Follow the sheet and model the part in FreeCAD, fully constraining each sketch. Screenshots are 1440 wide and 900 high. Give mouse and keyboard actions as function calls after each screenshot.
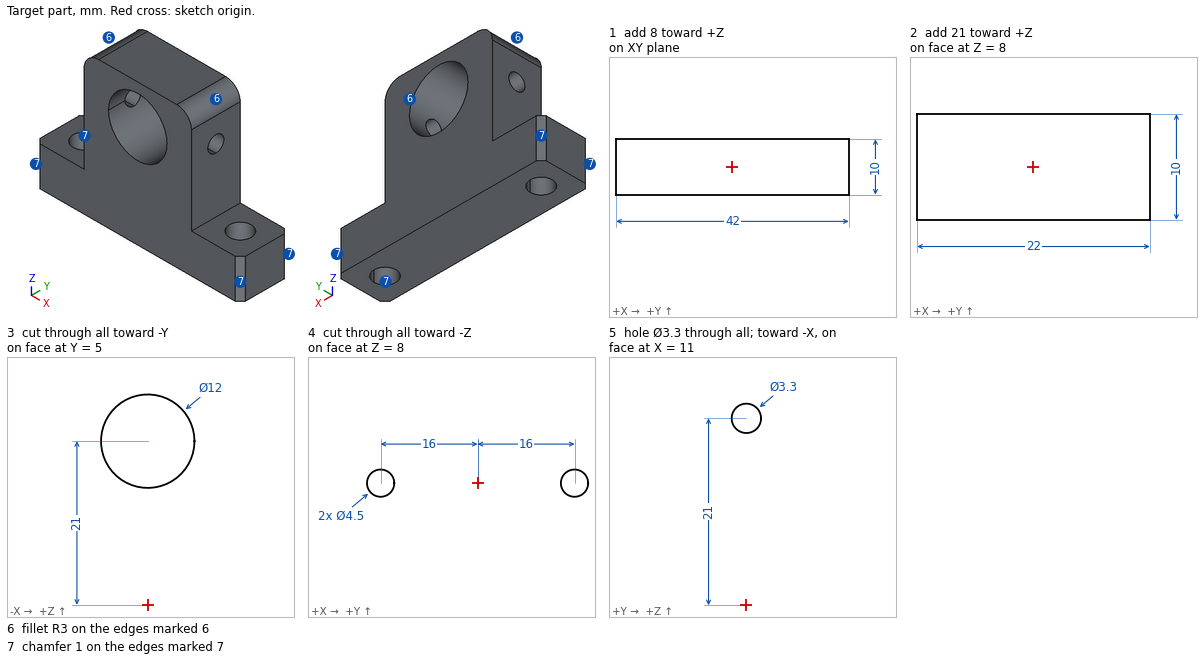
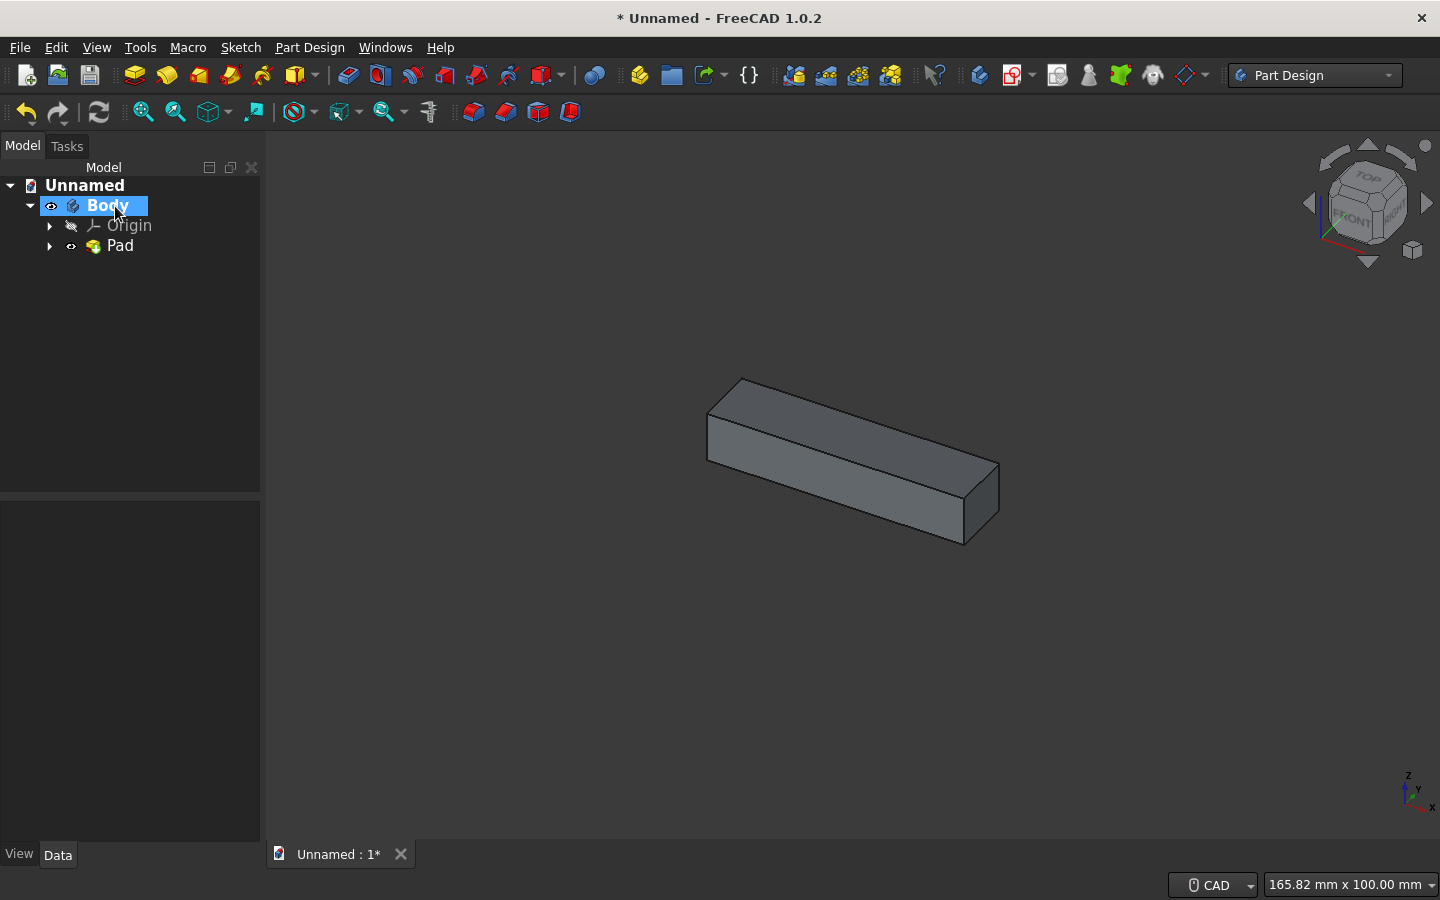
key(v)
key(f)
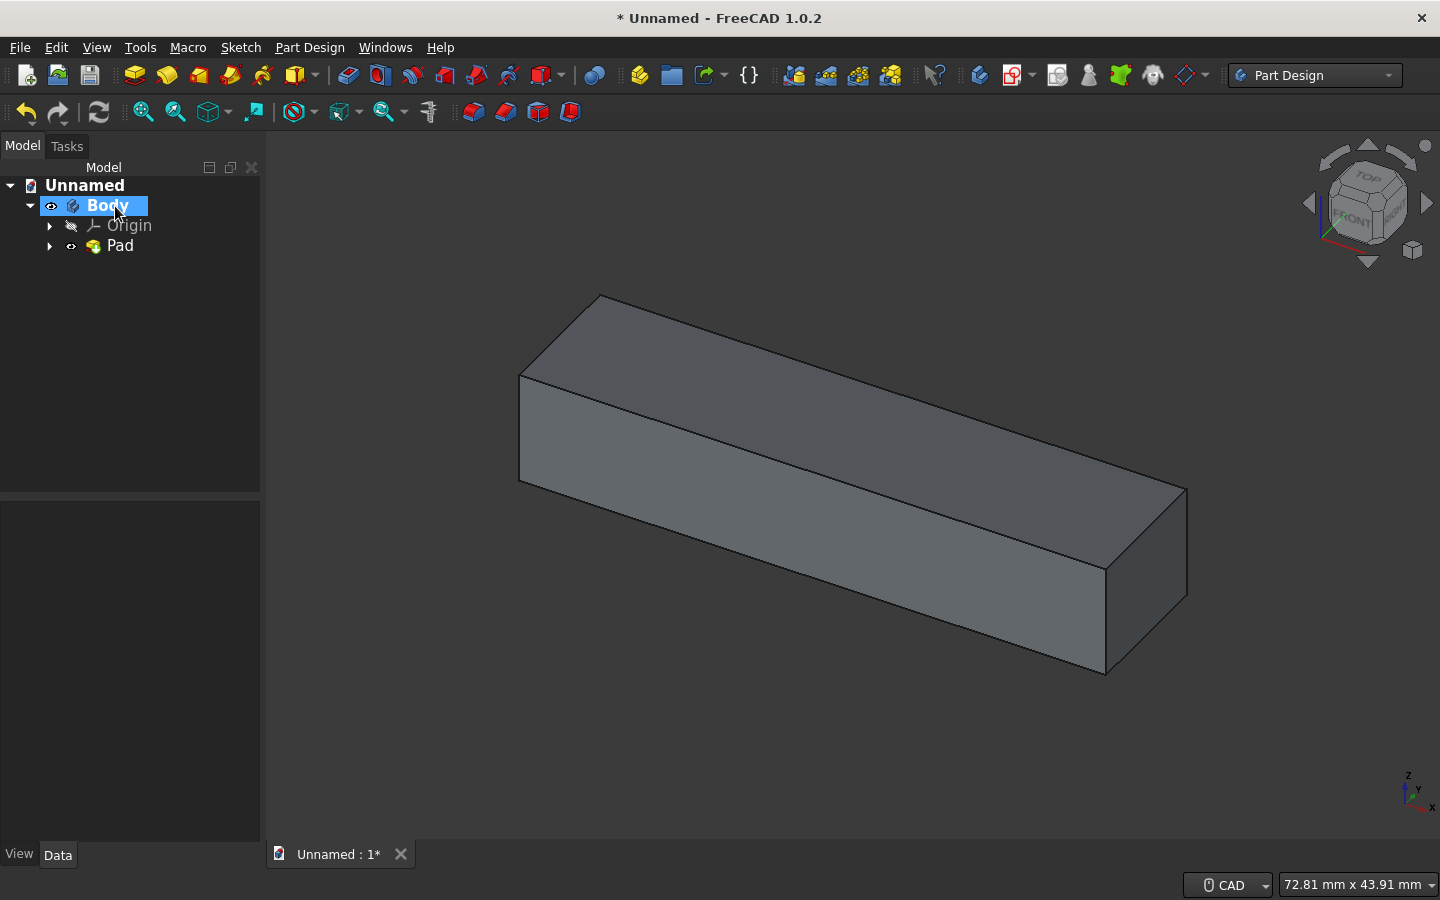
click(1021, 487)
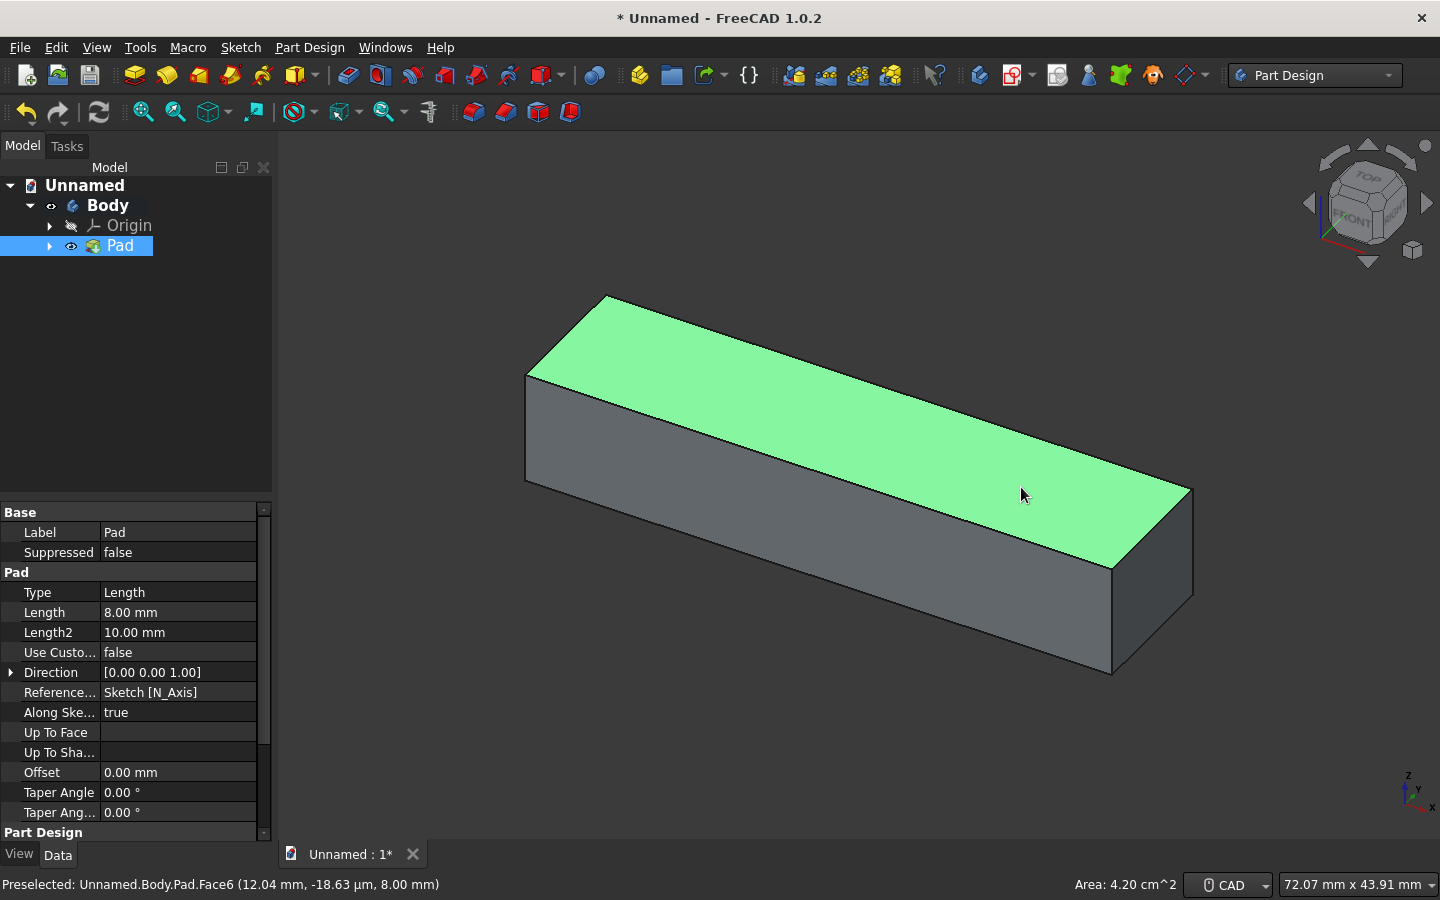
click(1012, 76)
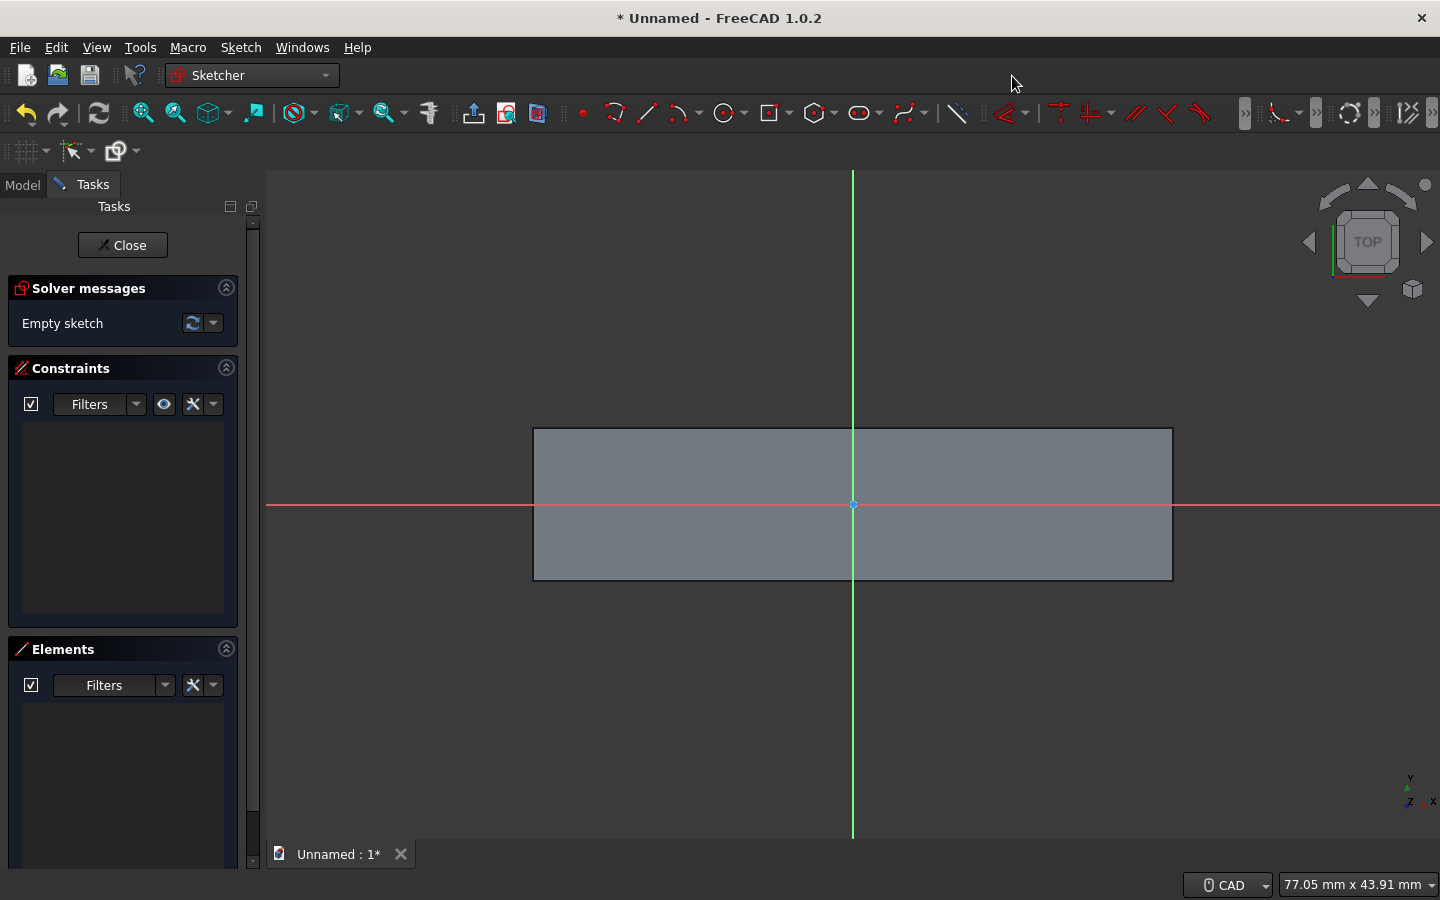
scroll(909, 504, up, 4)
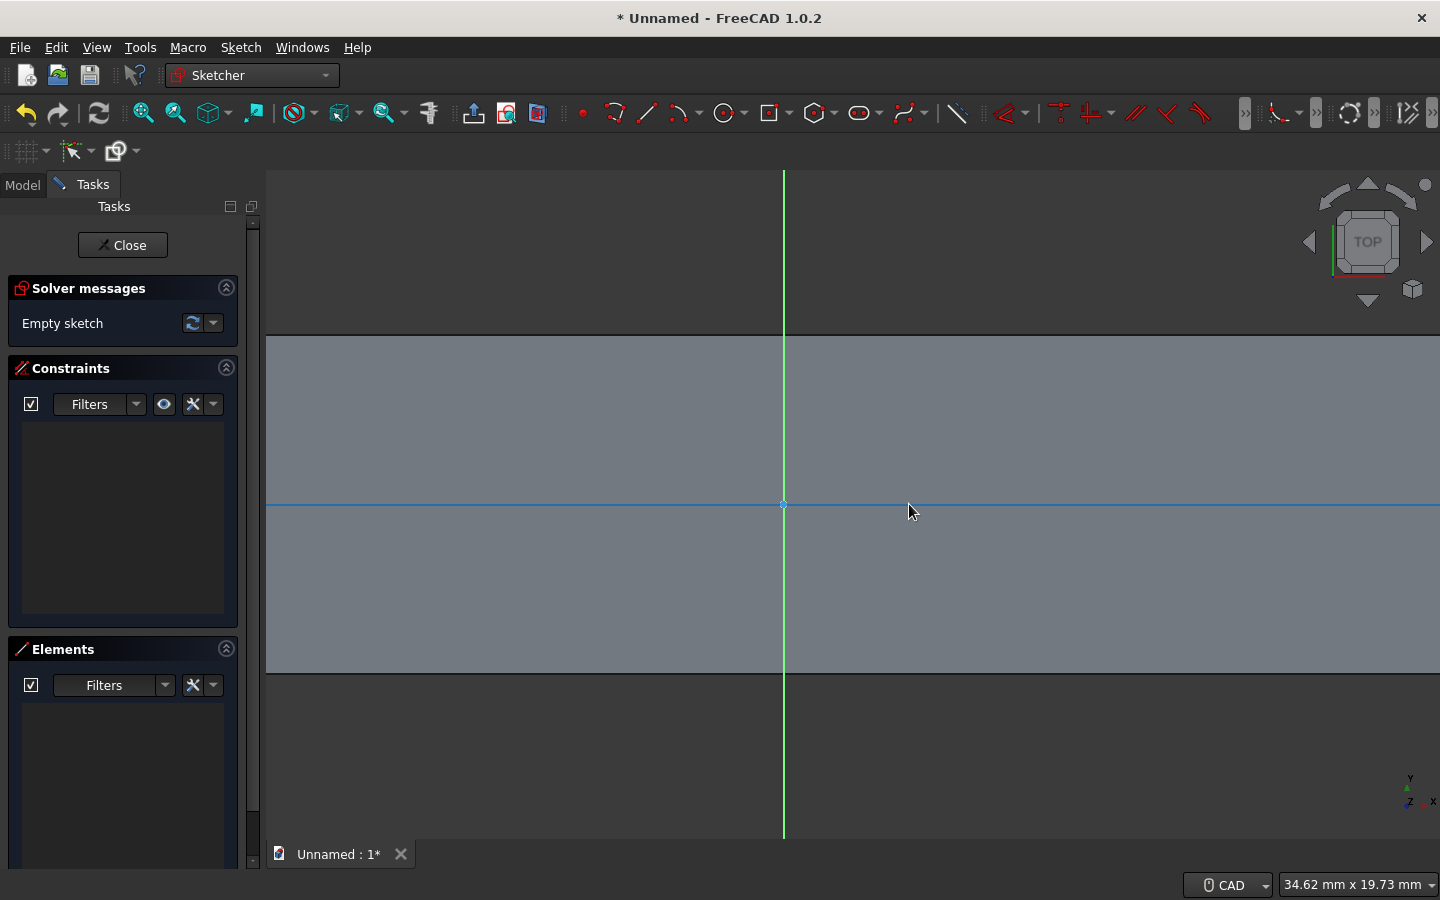
key(g)
key(v)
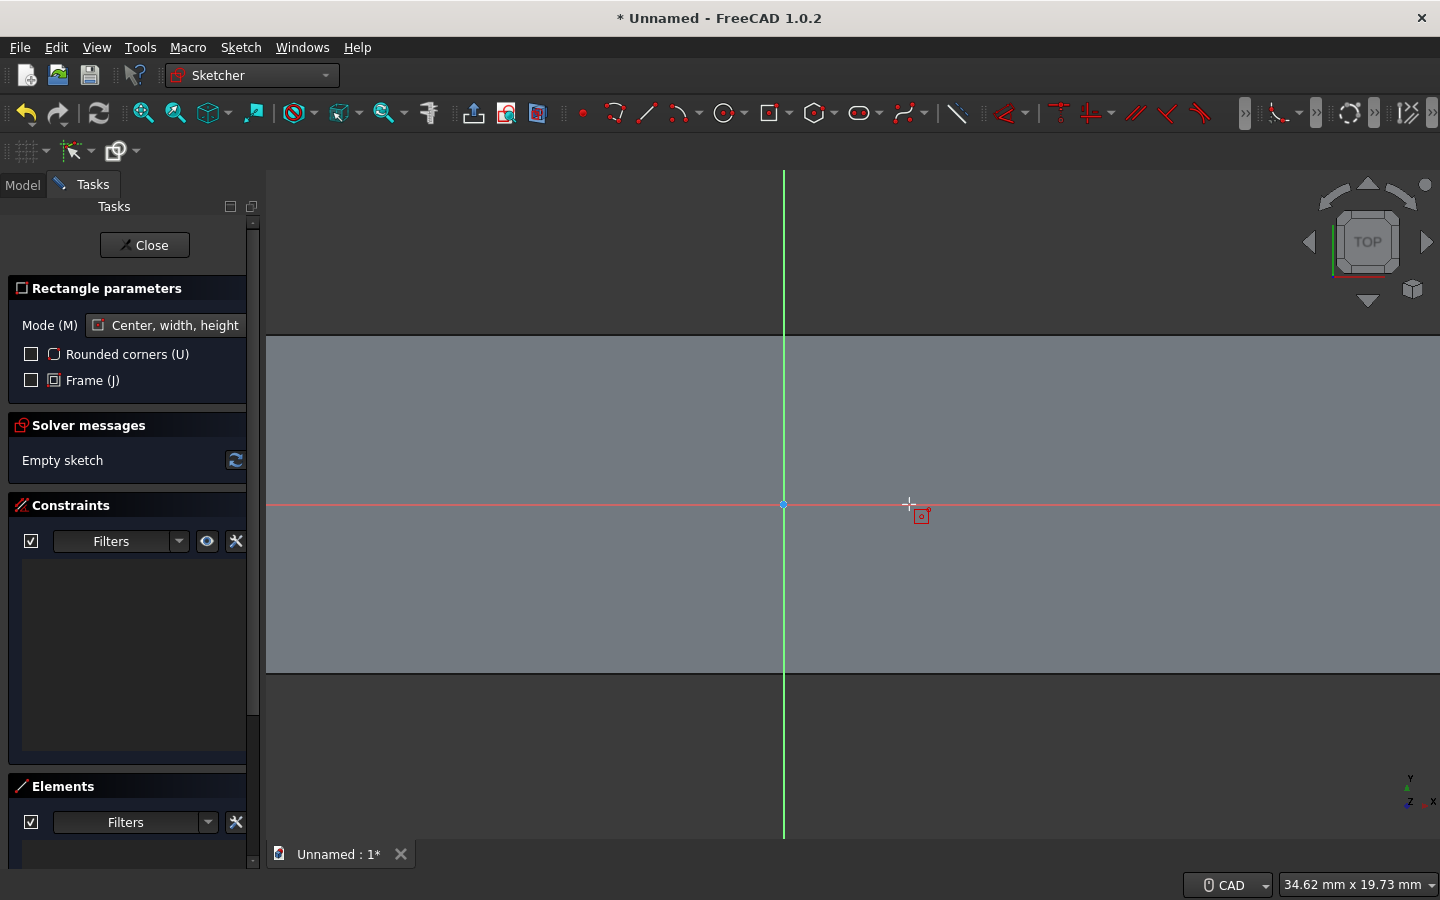
click(784, 504)
click(1157, 335)
key(Escape)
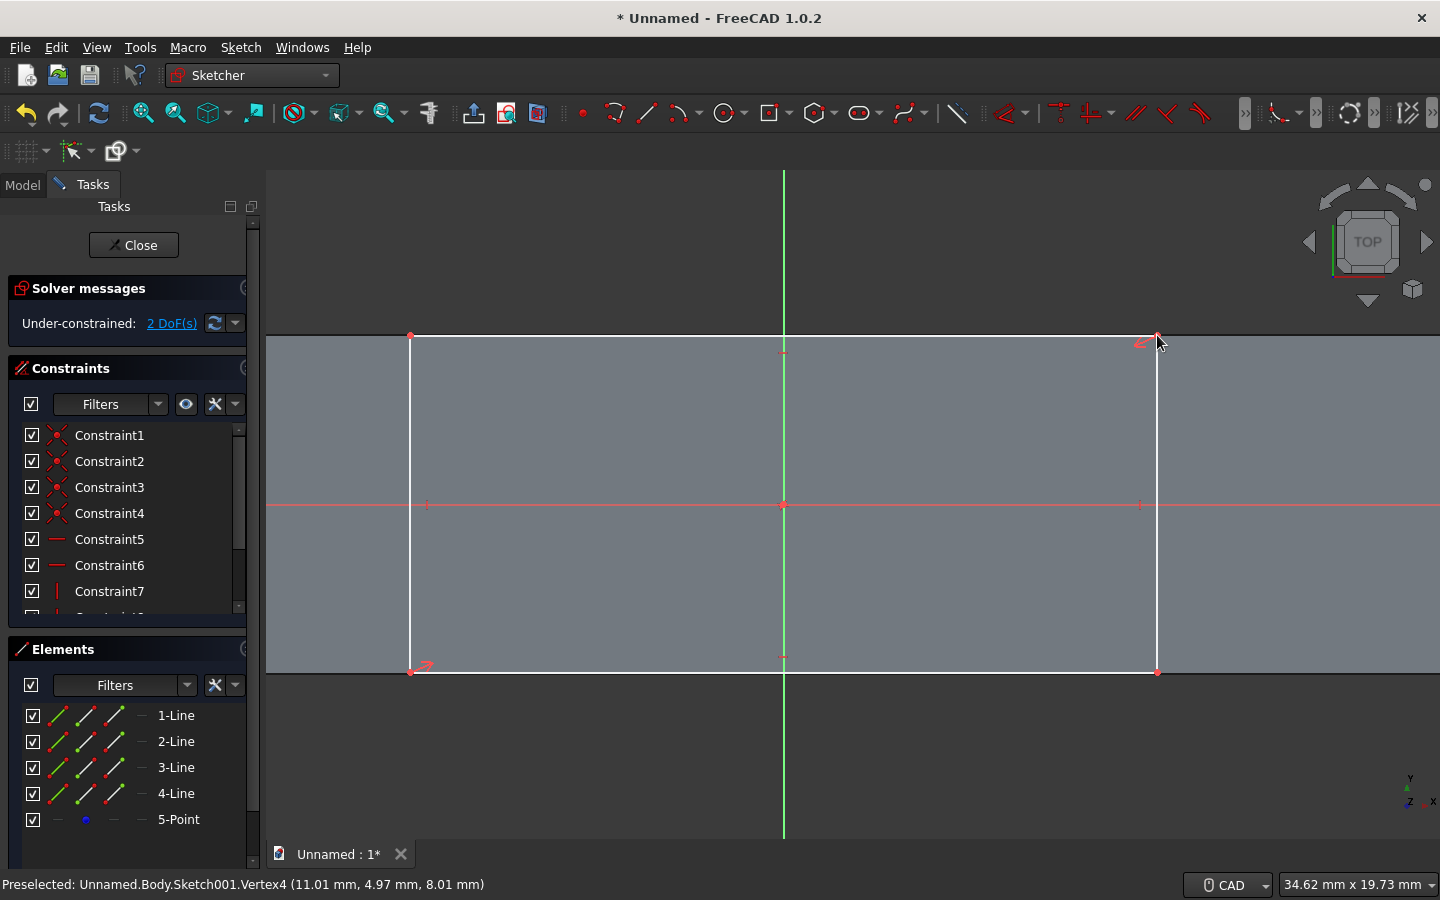
click(1004, 114)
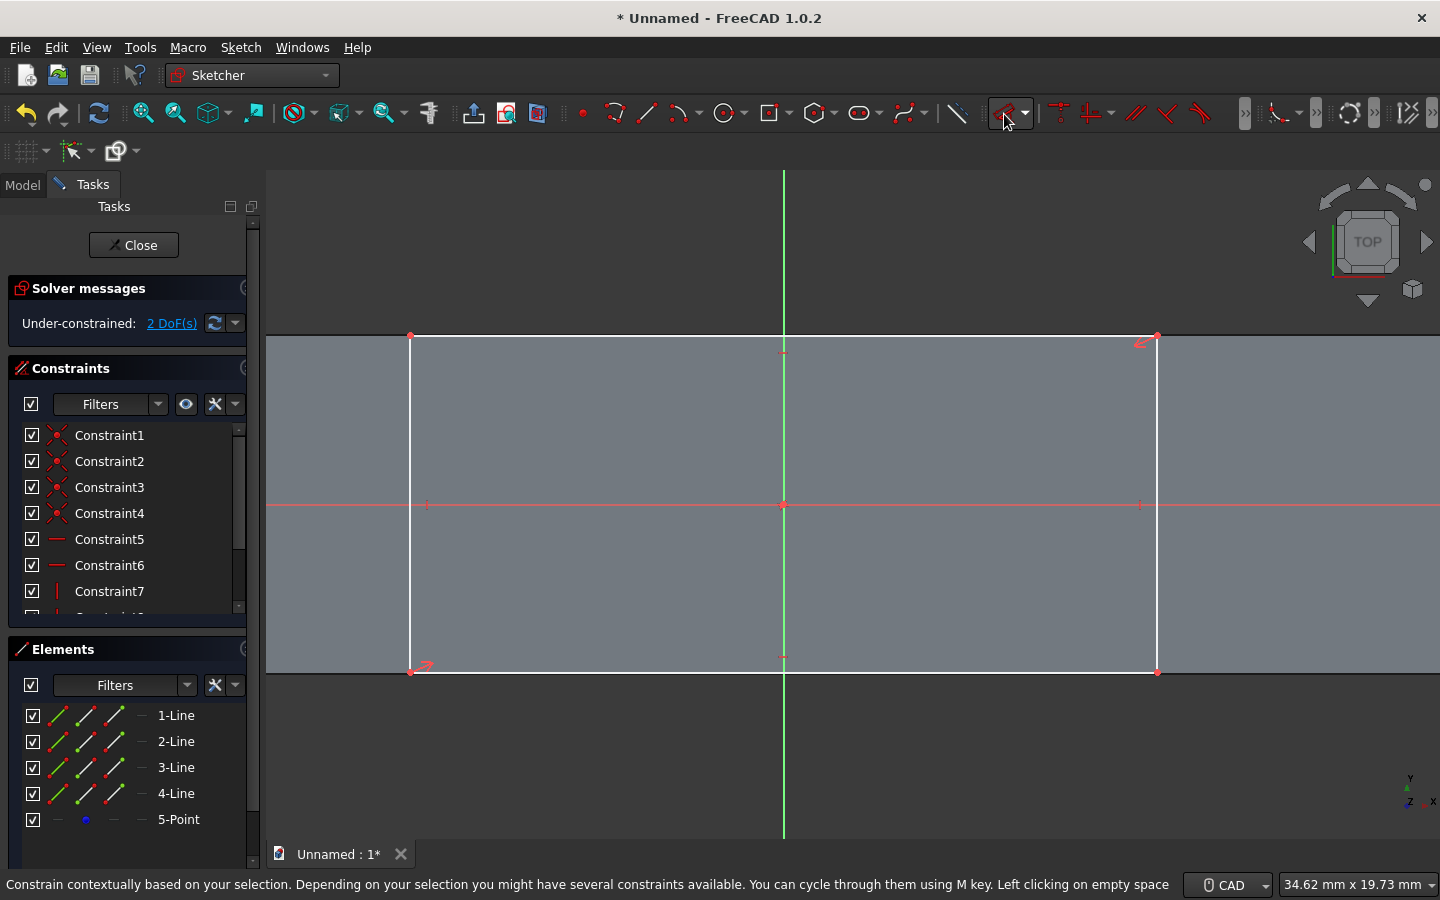
click(634, 673)
click(612, 707)